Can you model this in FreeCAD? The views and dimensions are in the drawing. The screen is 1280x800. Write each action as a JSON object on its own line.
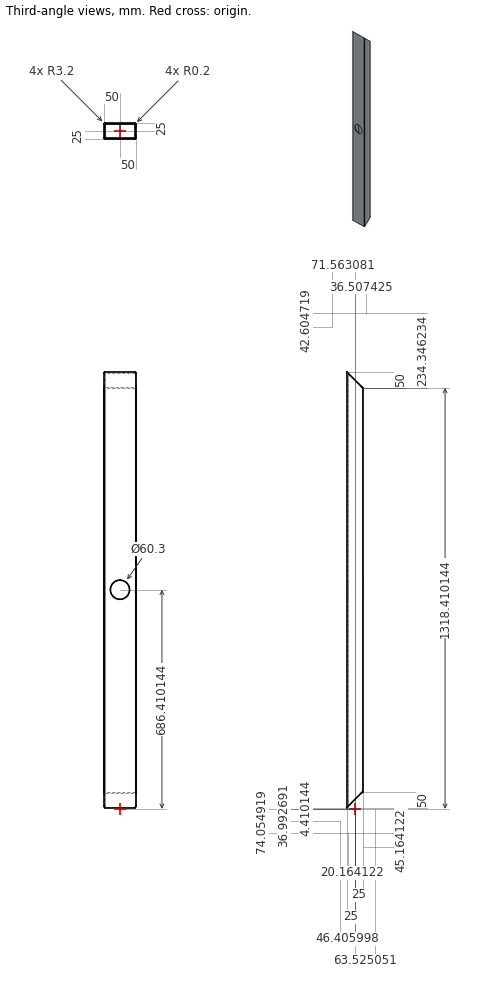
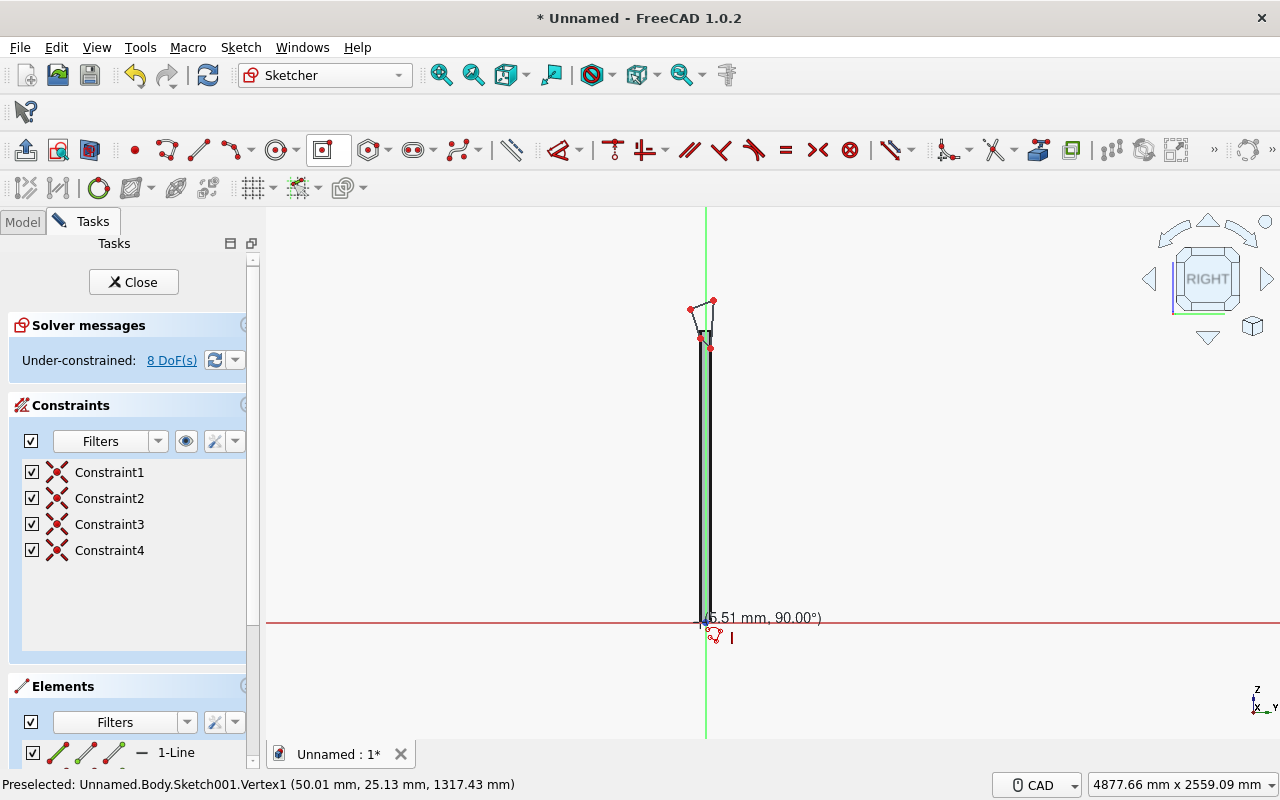
{"action": "scroll", "coordinate": [696, 630], "scroll_direction": "up", "scroll_amount": 4}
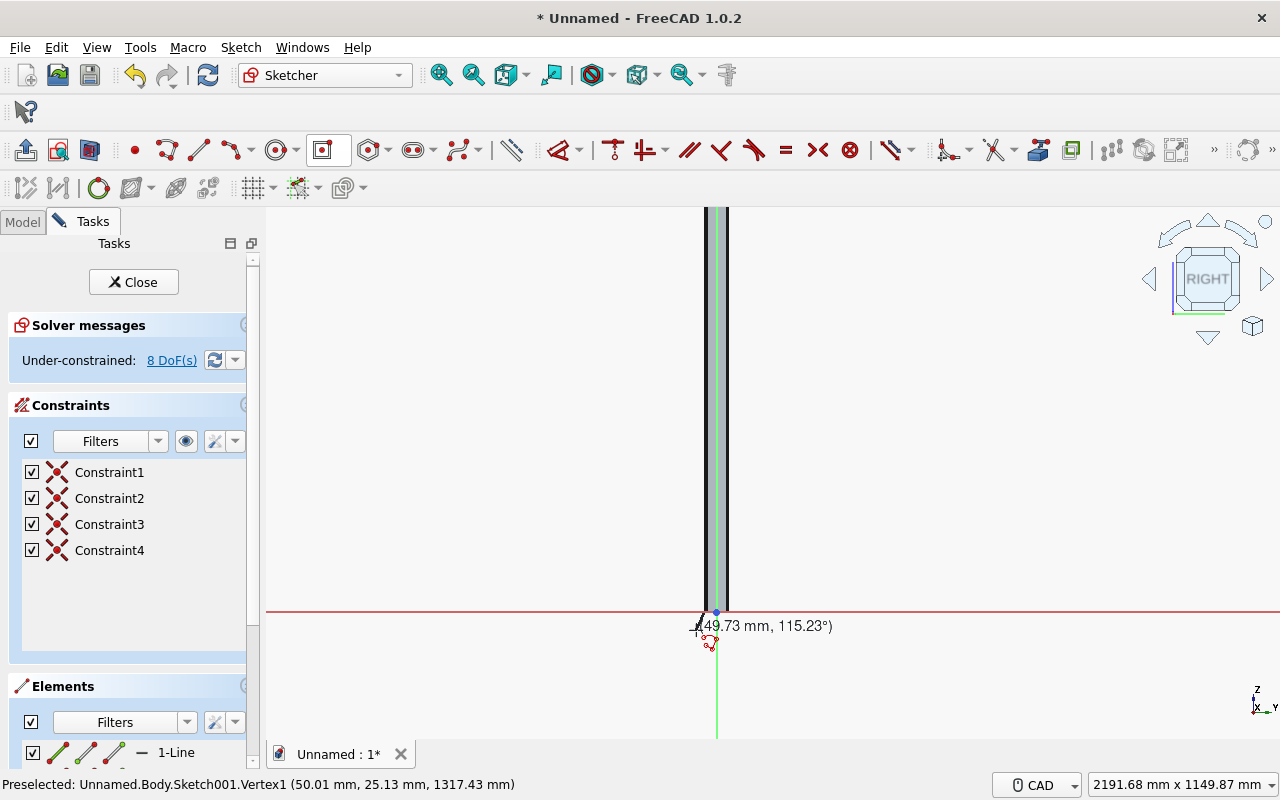
{"action": "left_click", "coordinate": [695, 629]}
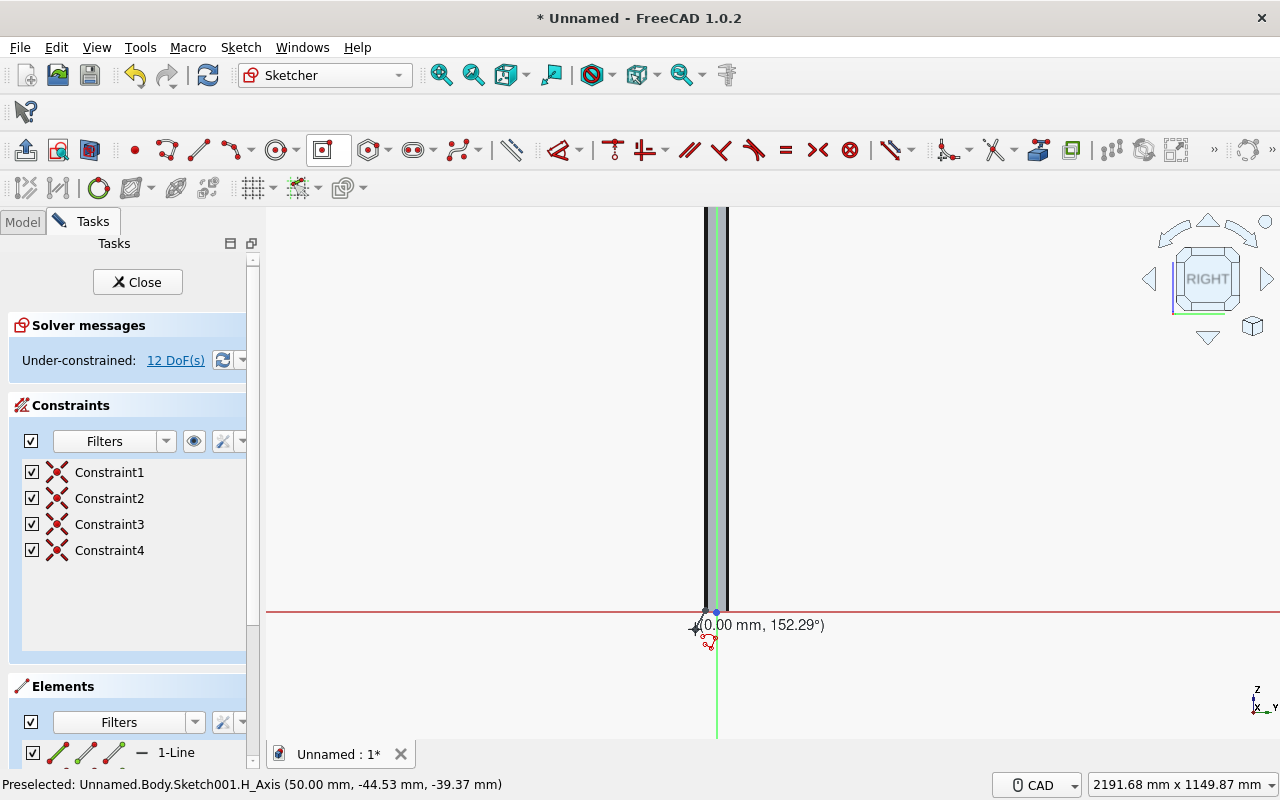
{"action": "scroll", "coordinate": [707, 647], "scroll_direction": "up", "scroll_amount": 3}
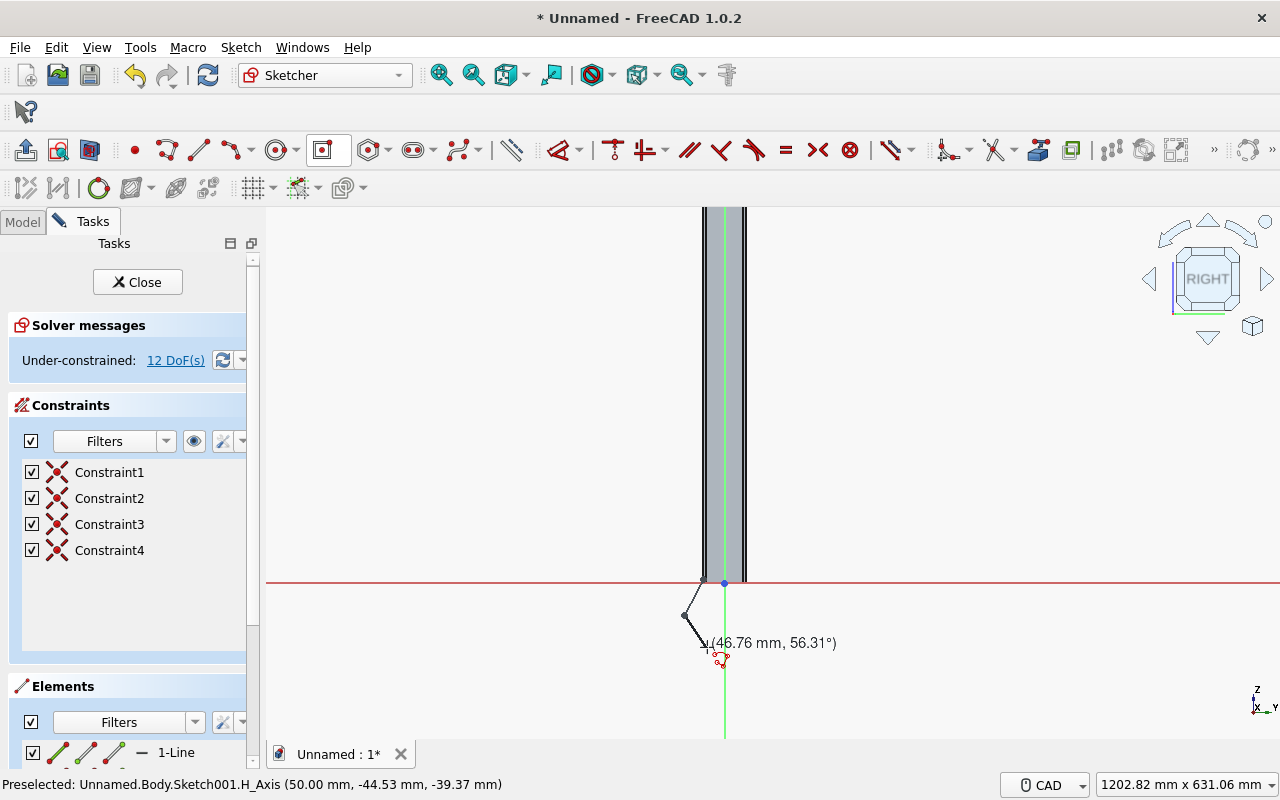
{"action": "left_click", "coordinate": [708, 646]}
{"action": "left_click", "coordinate": [746, 684]}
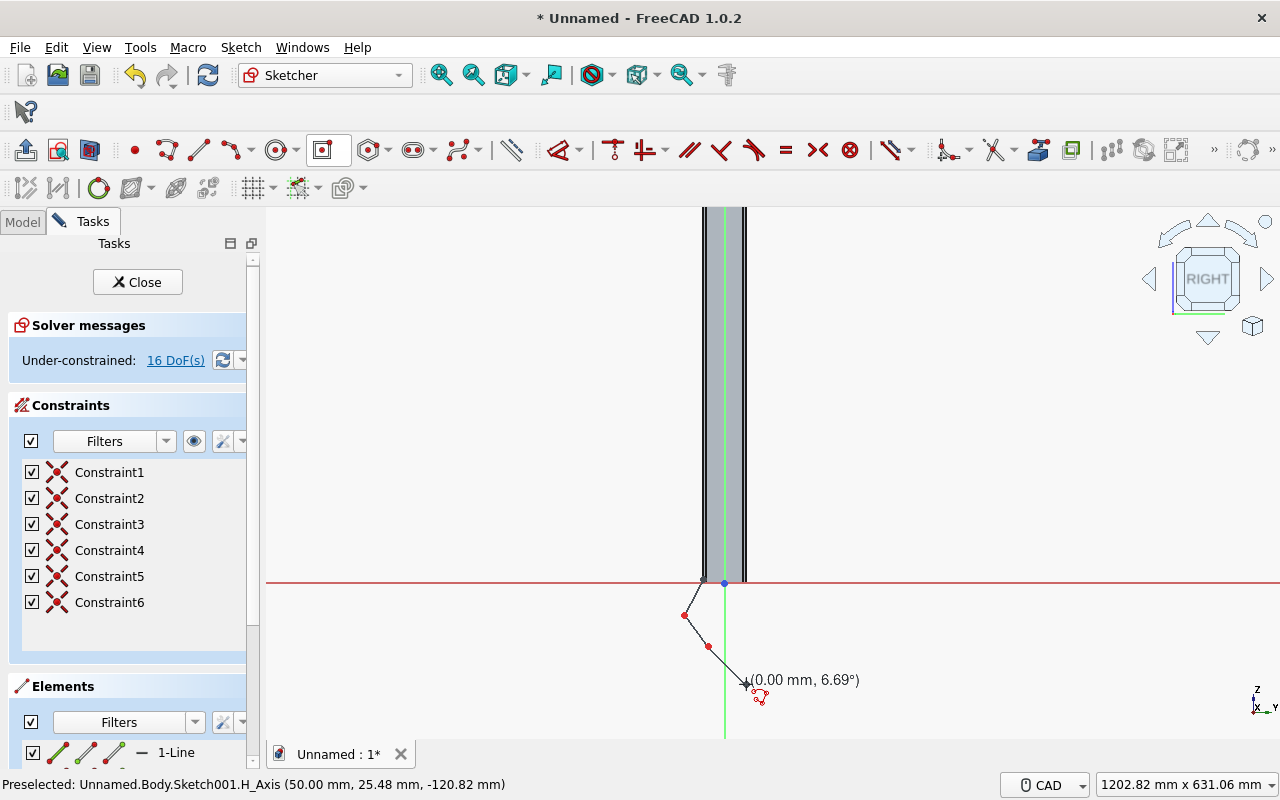
{"action": "scroll", "coordinate": [699, 635], "scroll_direction": "down", "scroll_amount": 7}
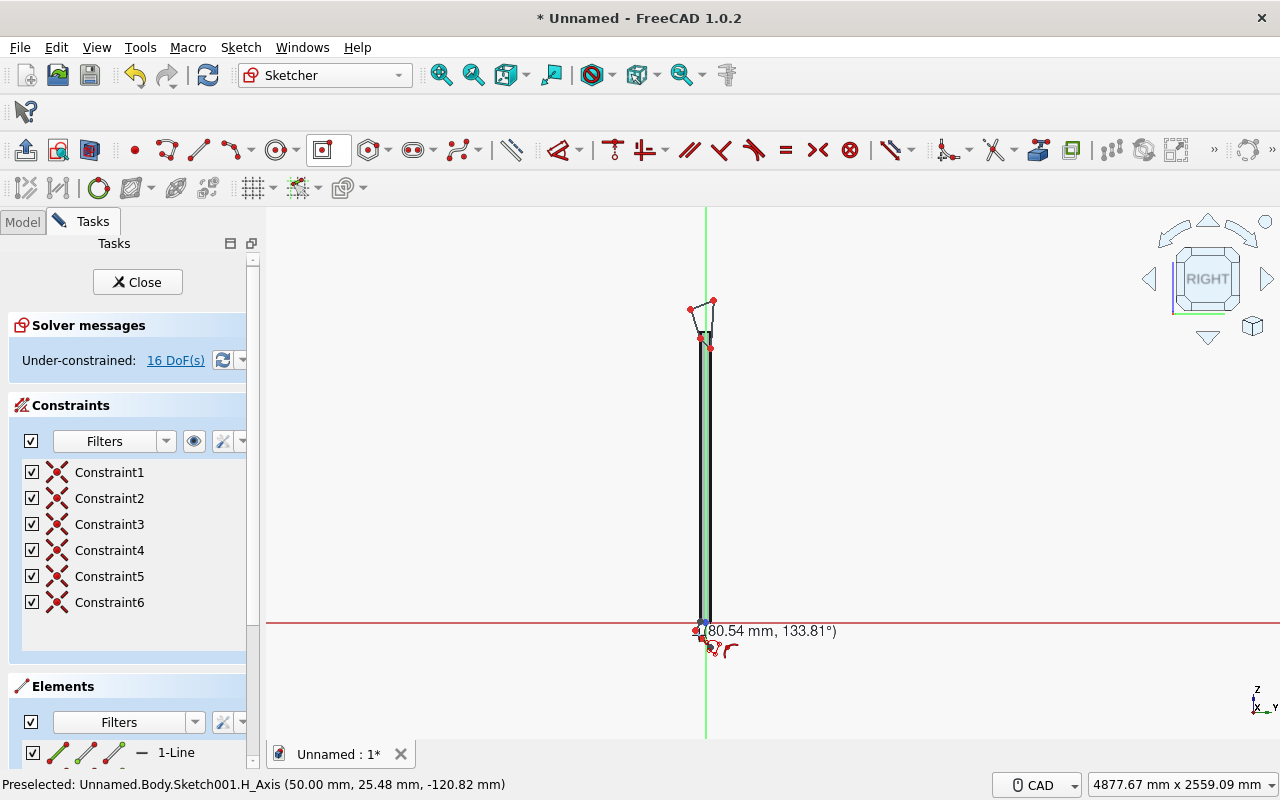
{"action": "left_click", "coordinate": [719, 623]}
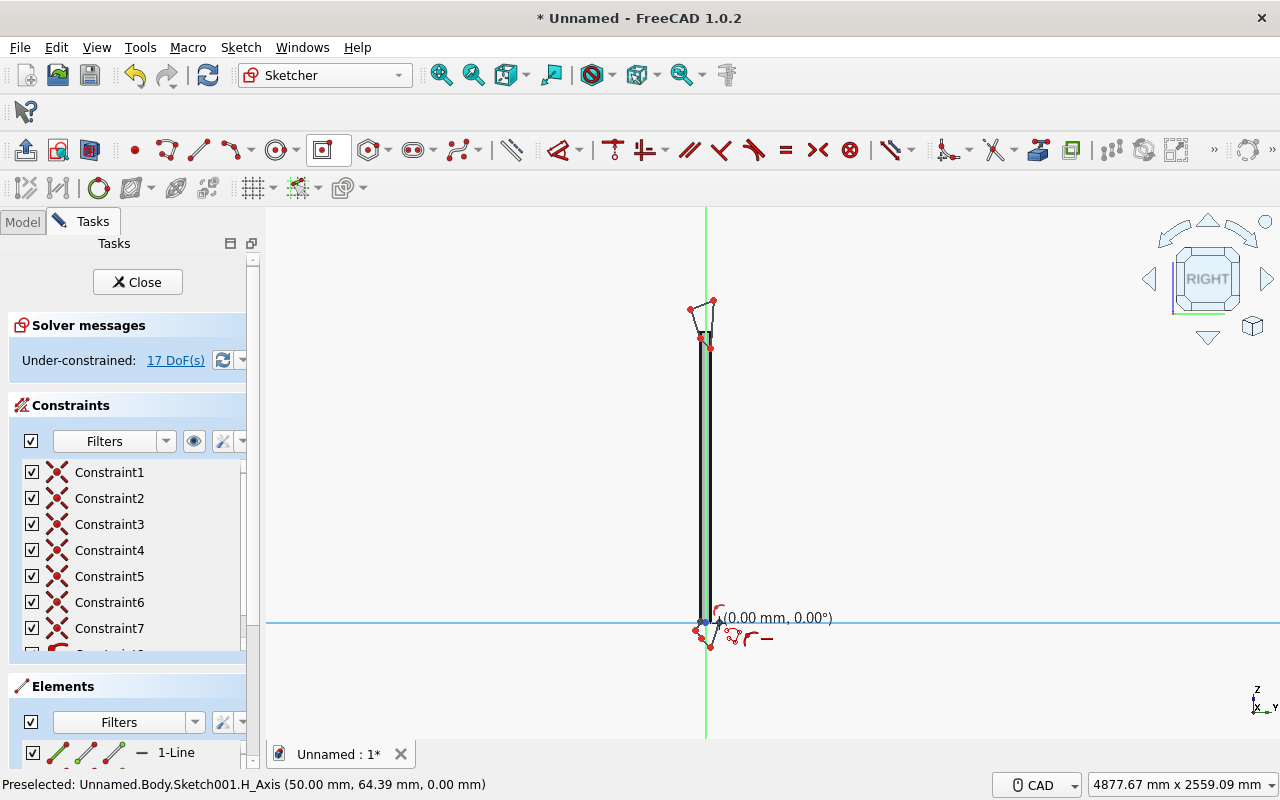
{"action": "scroll", "coordinate": [711, 612], "scroll_direction": "up", "scroll_amount": 6}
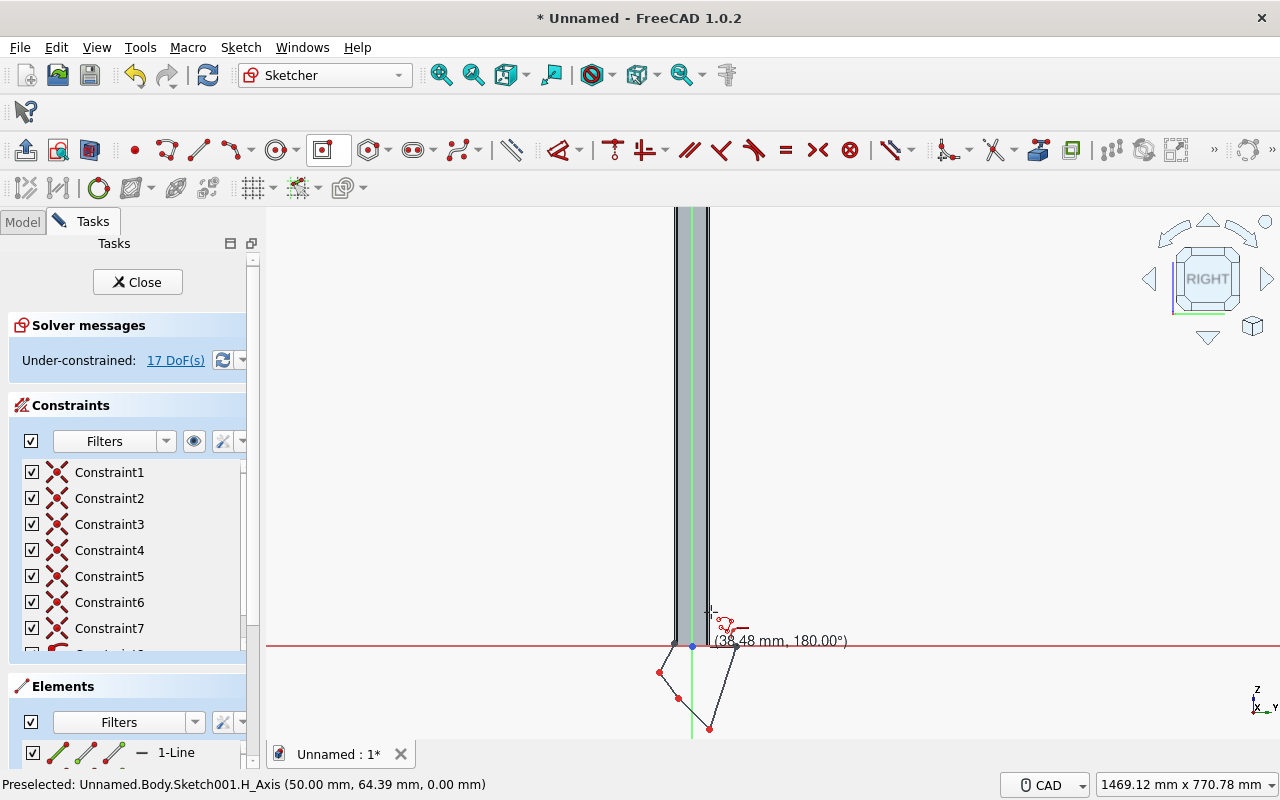
{"action": "left_click", "coordinate": [709, 609]}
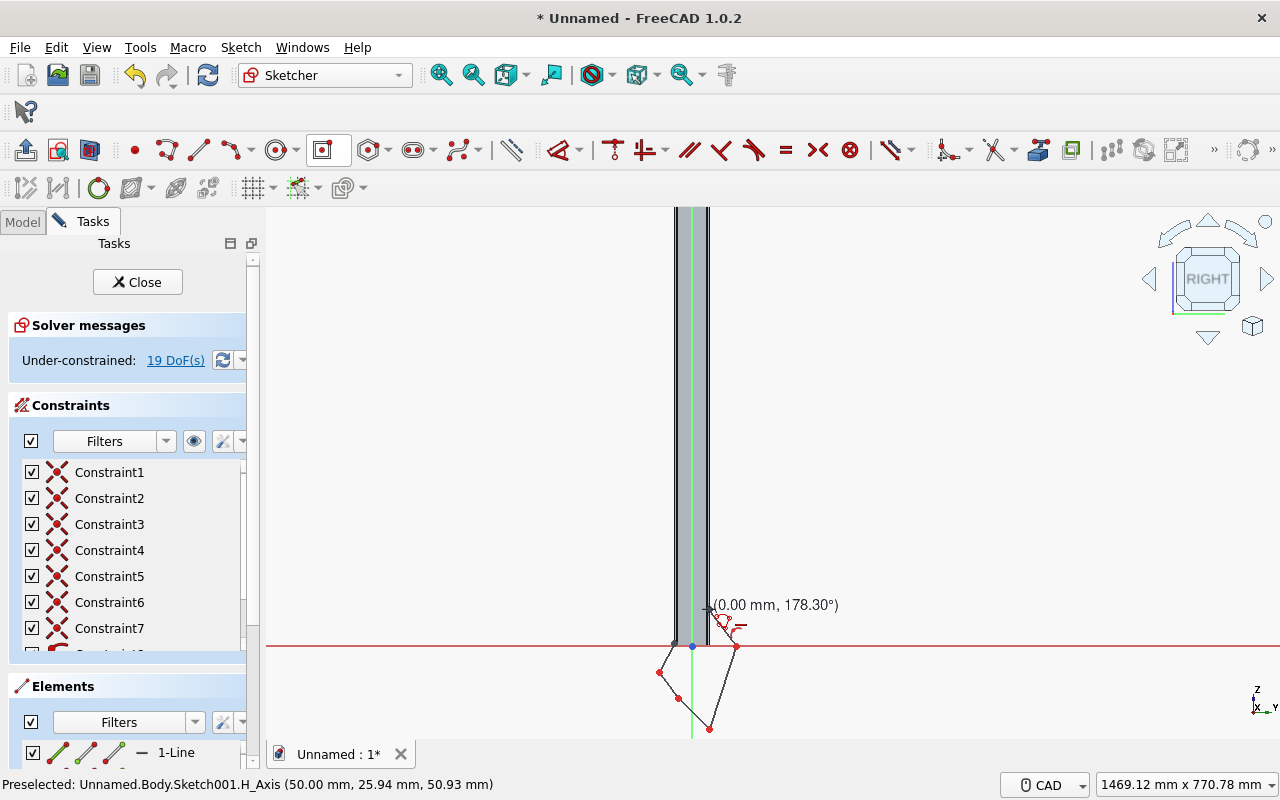
{"action": "scroll", "coordinate": [675, 643], "scroll_direction": "up", "scroll_amount": 9}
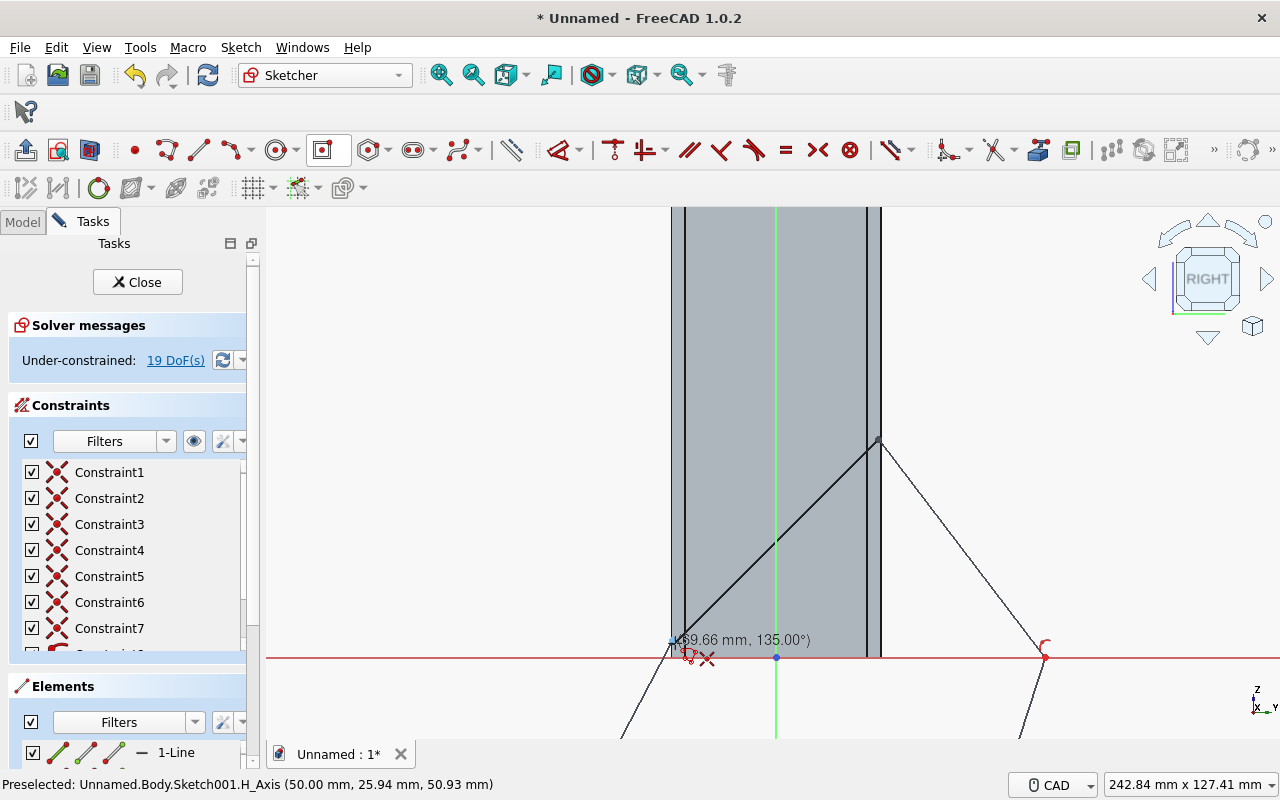
{"action": "left_click", "coordinate": [672, 641]}
{"action": "key", "text": "Escape"}
{"action": "key", "text": "Escape"}